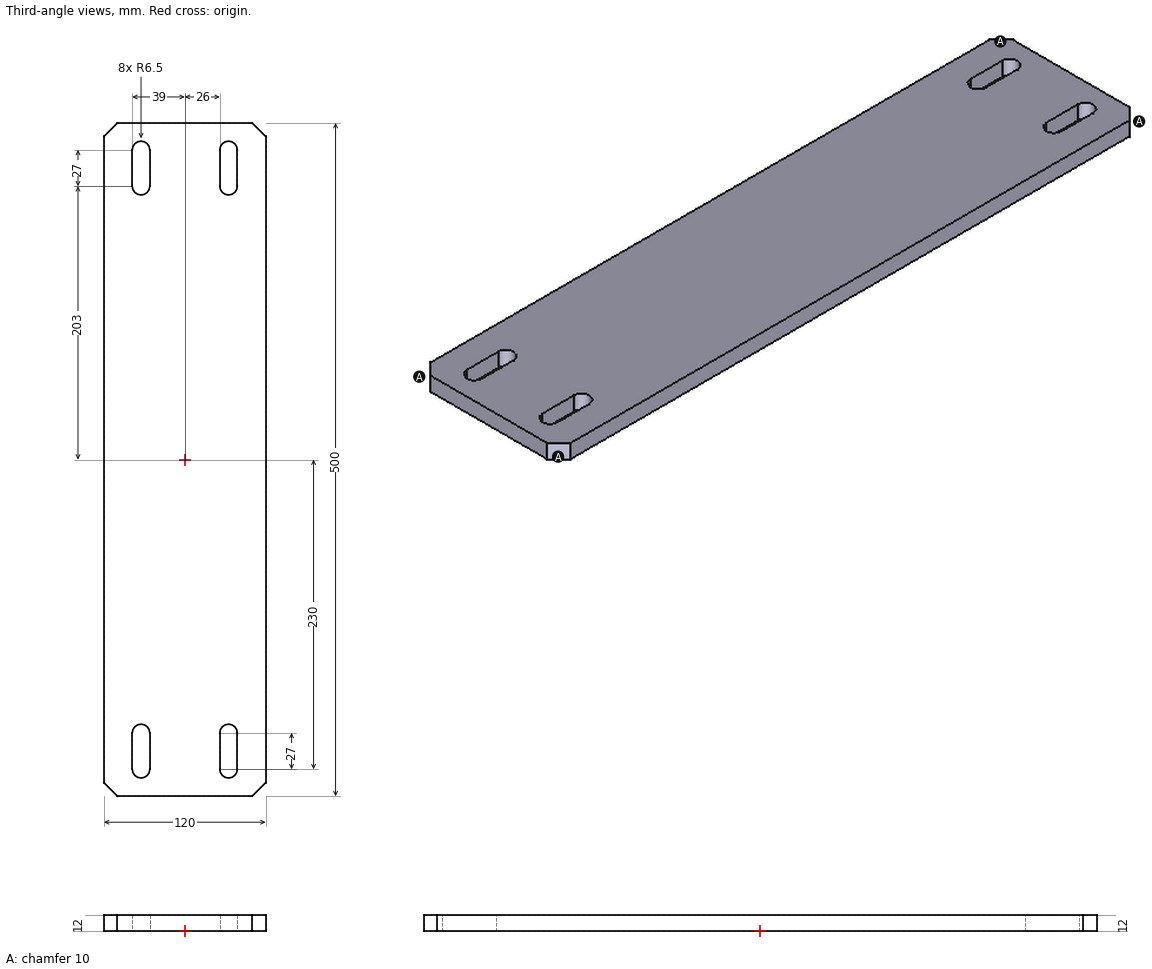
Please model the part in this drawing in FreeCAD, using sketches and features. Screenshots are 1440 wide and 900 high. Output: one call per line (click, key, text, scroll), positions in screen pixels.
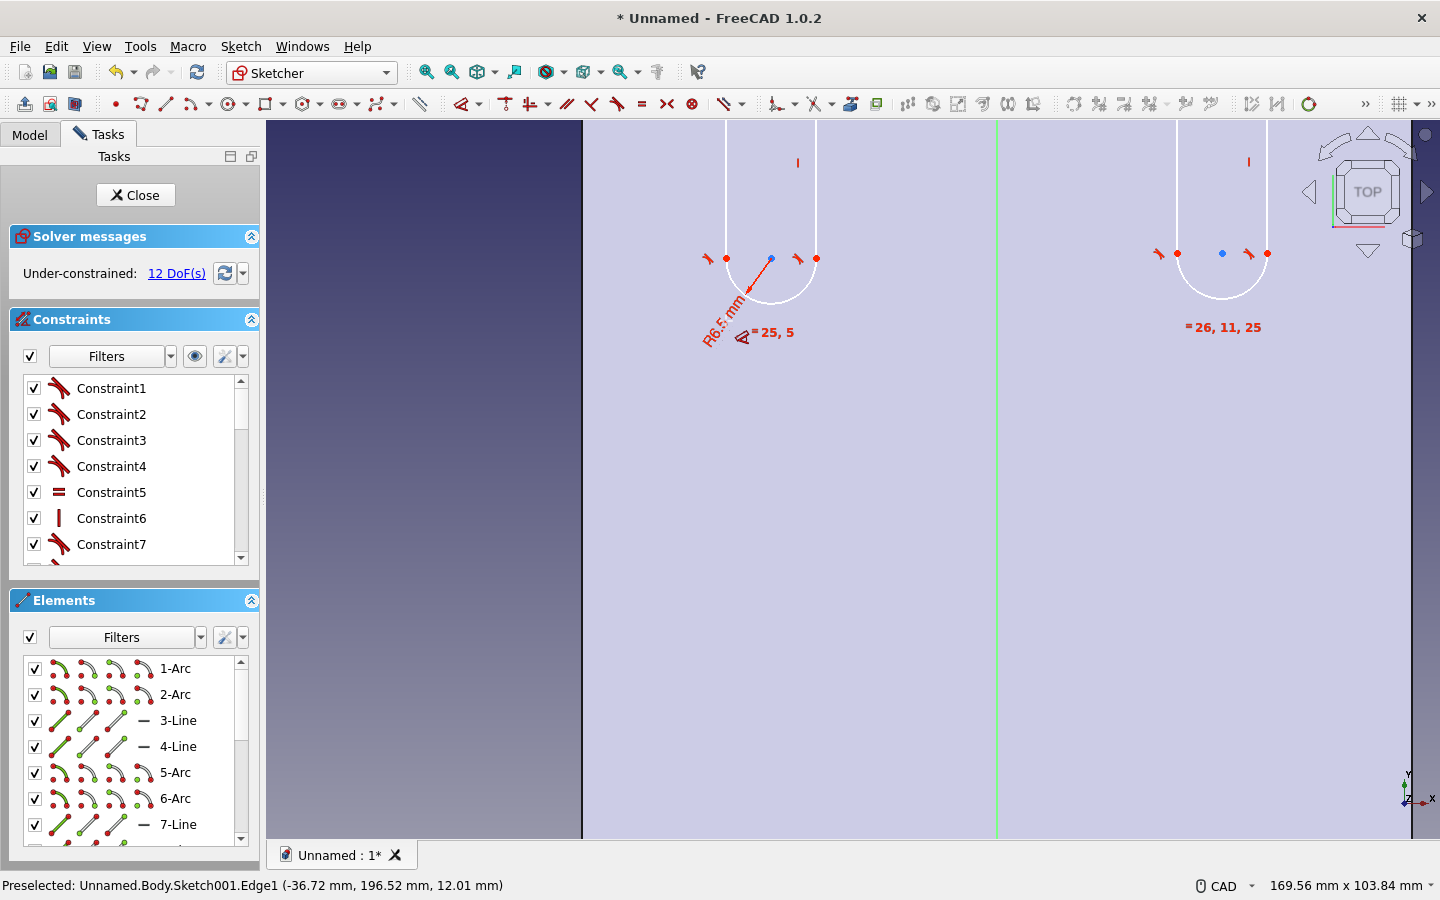
scroll(751, 296, down, 10)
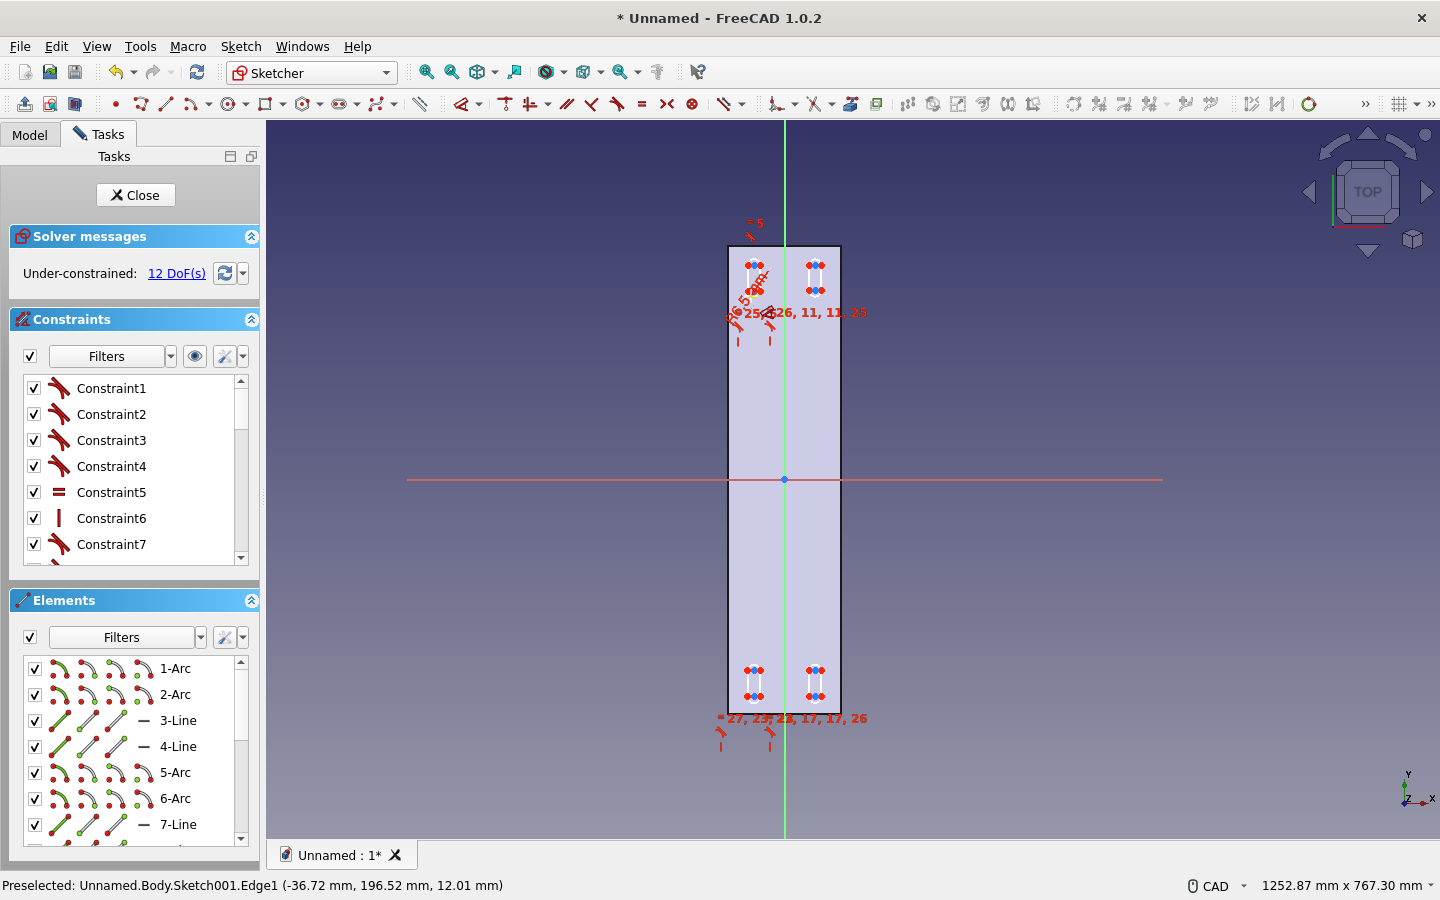
scroll(748, 283, up, 3)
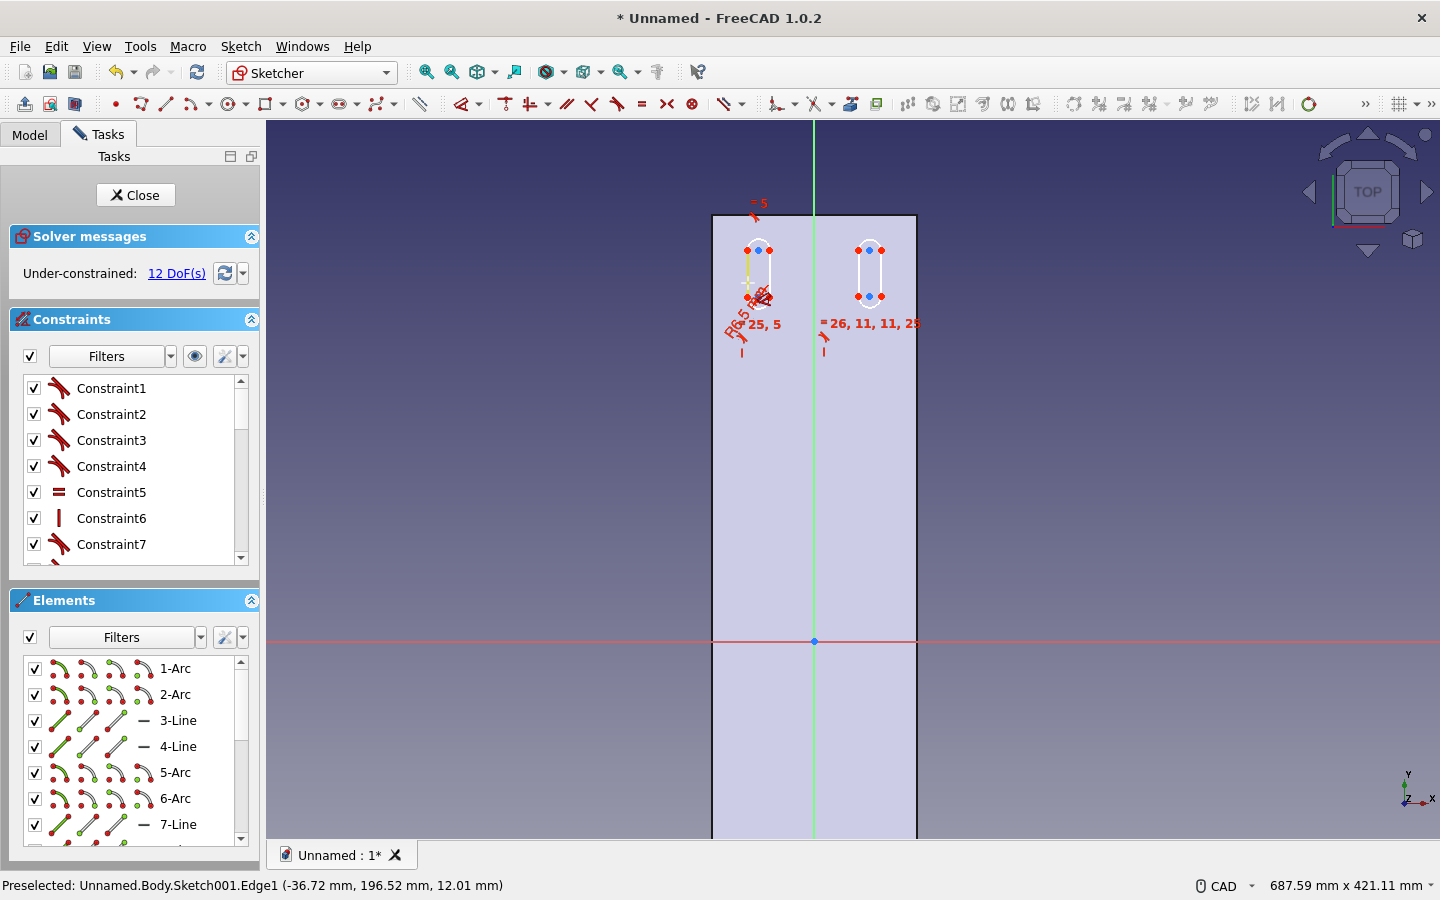
click(748, 283)
click(714, 274)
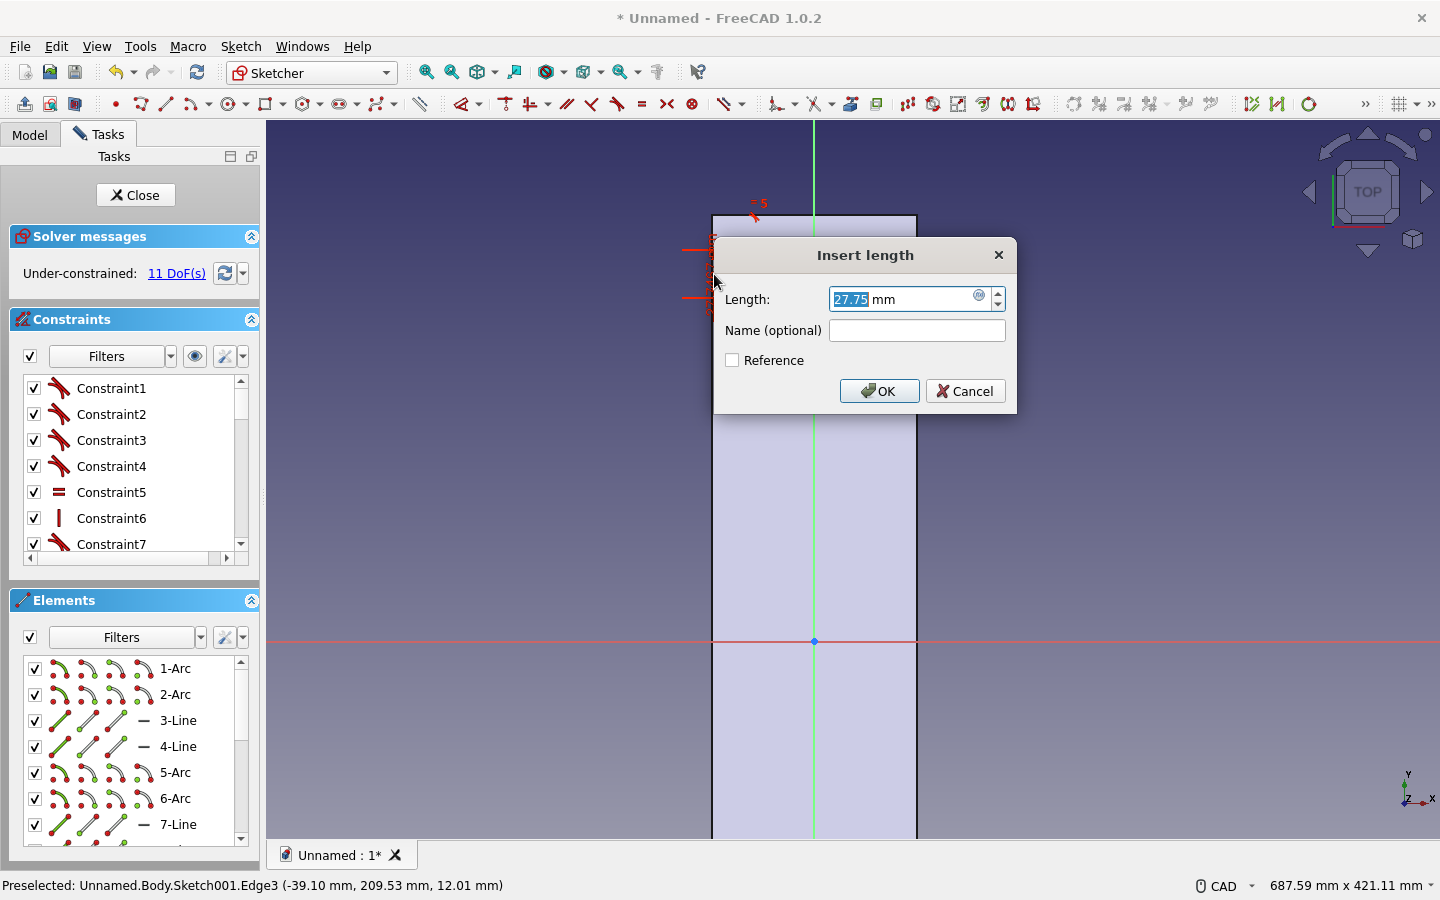
text(27)
key(Return)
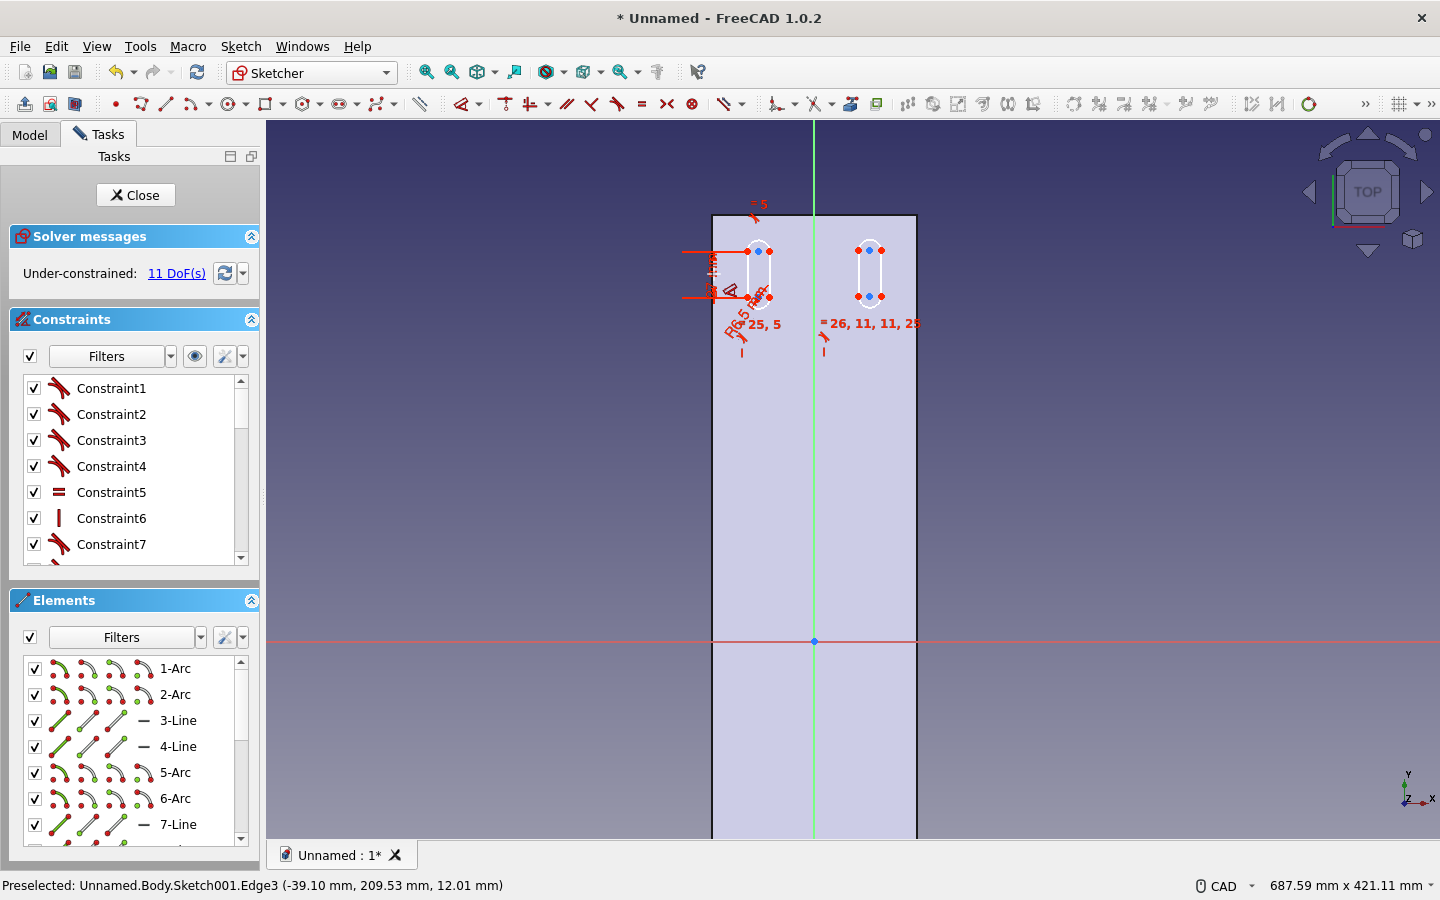
click(859, 283)
click(917, 274)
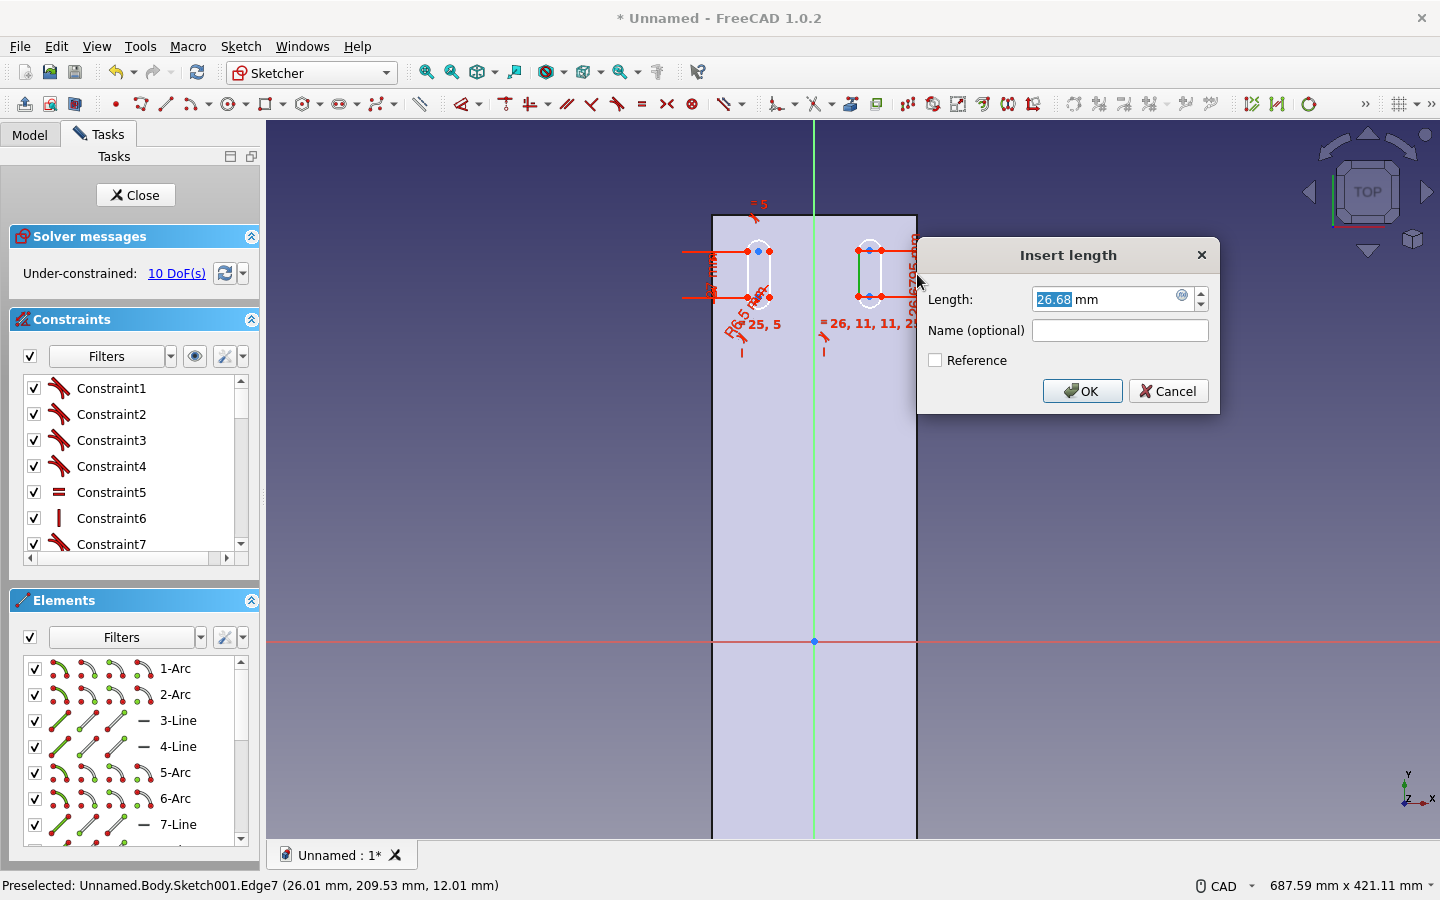
text(27)
key(Return)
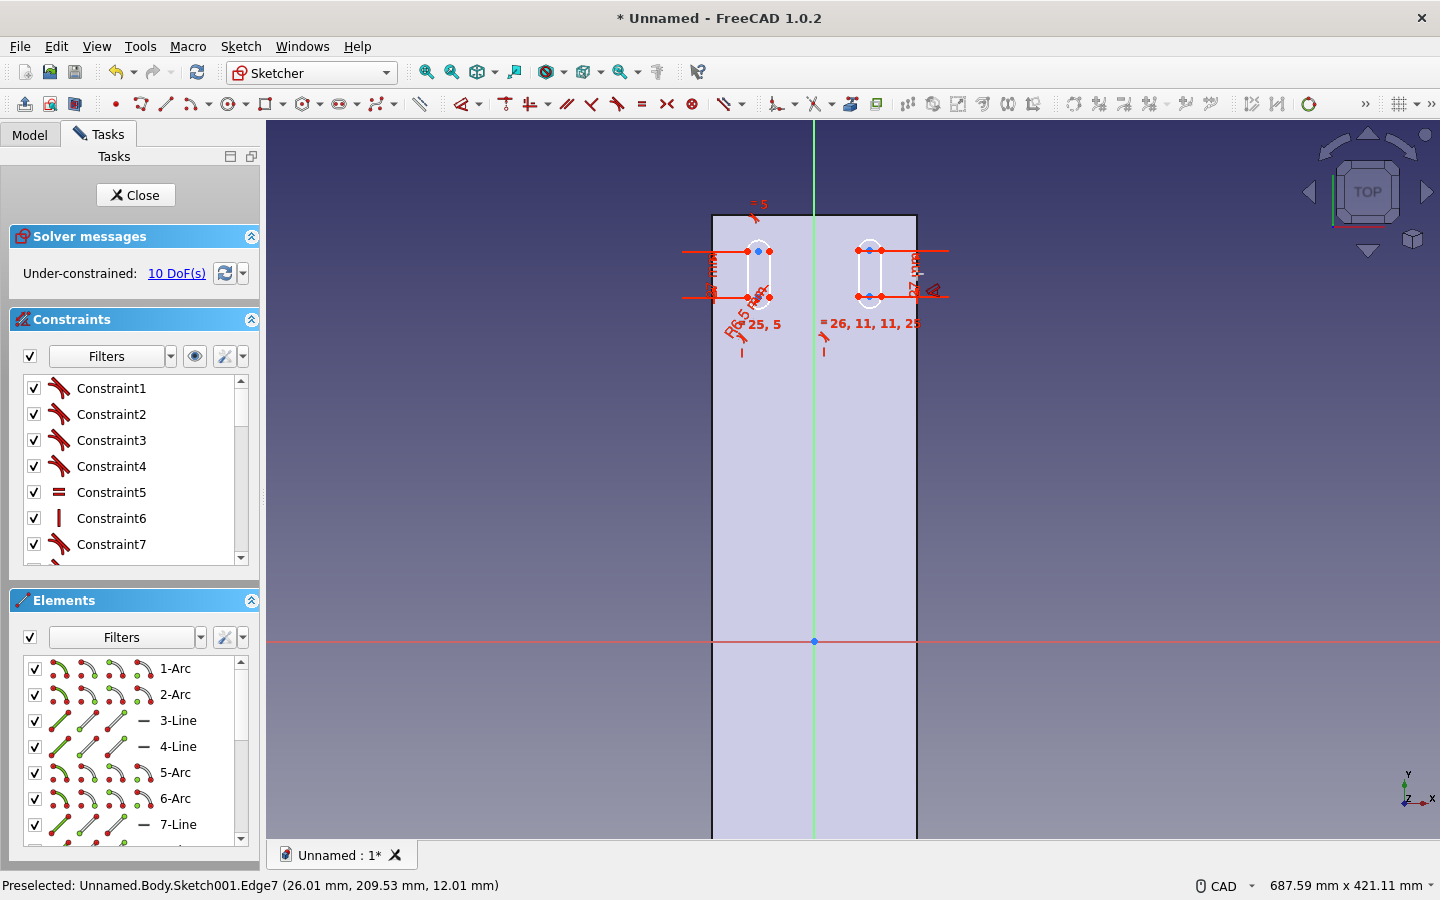
scroll(748, 282, down, 3)